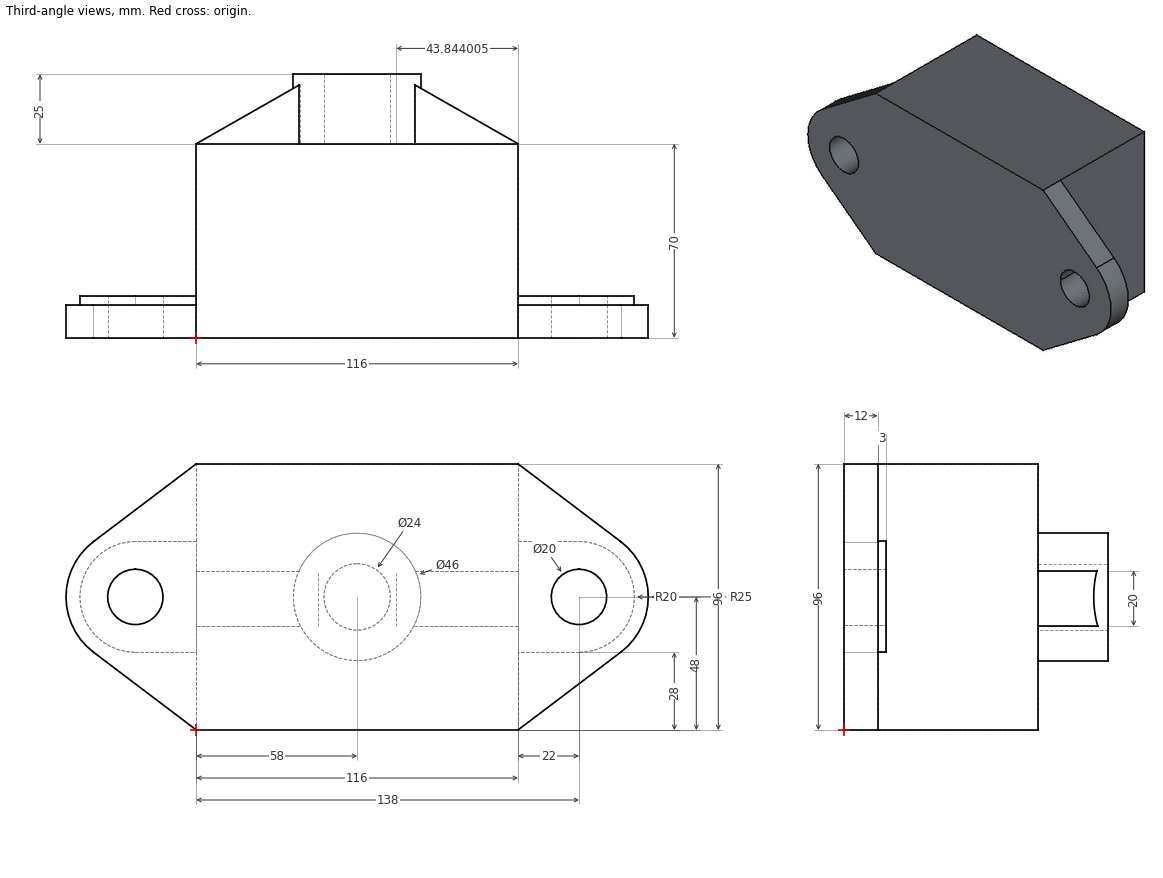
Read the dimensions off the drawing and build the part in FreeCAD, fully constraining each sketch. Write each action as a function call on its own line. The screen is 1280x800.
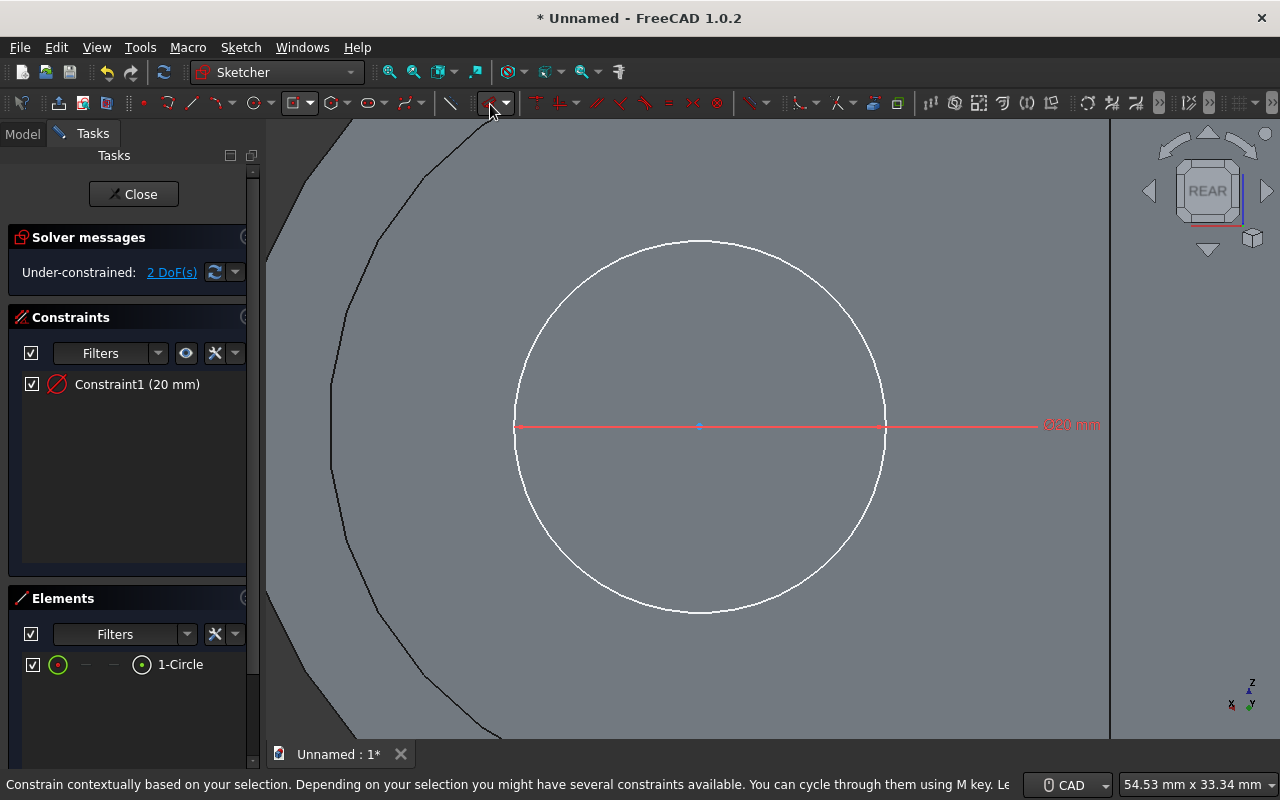
click(700, 427)
click(666, 569)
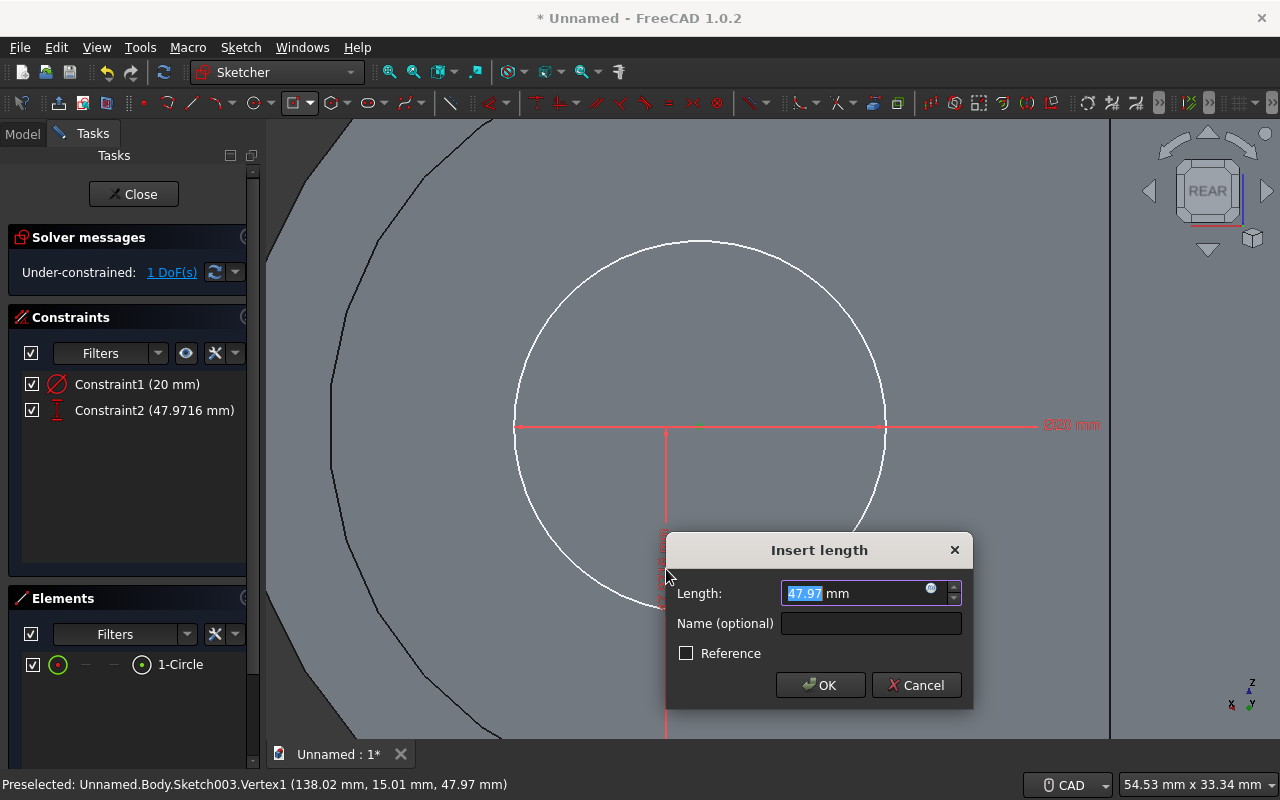
text(48)
key(Return)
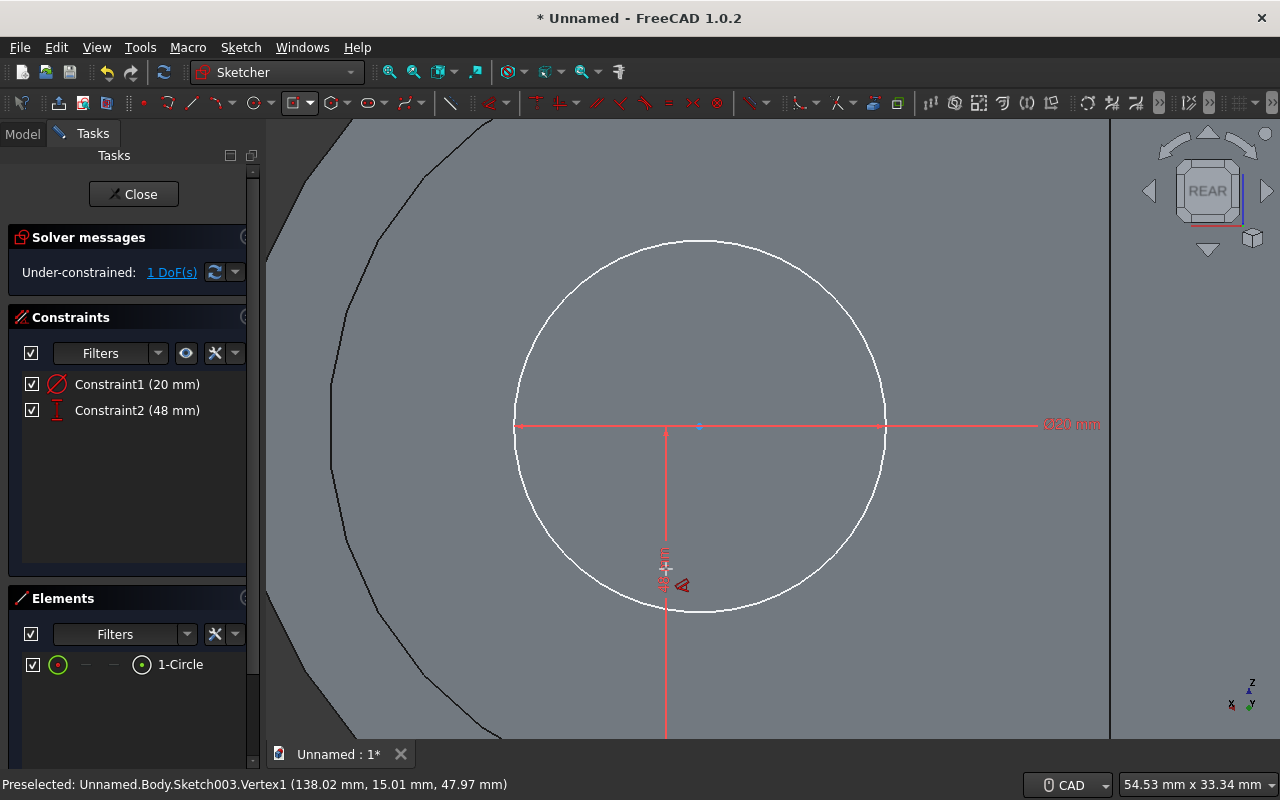
click(700, 426)
click(908, 392)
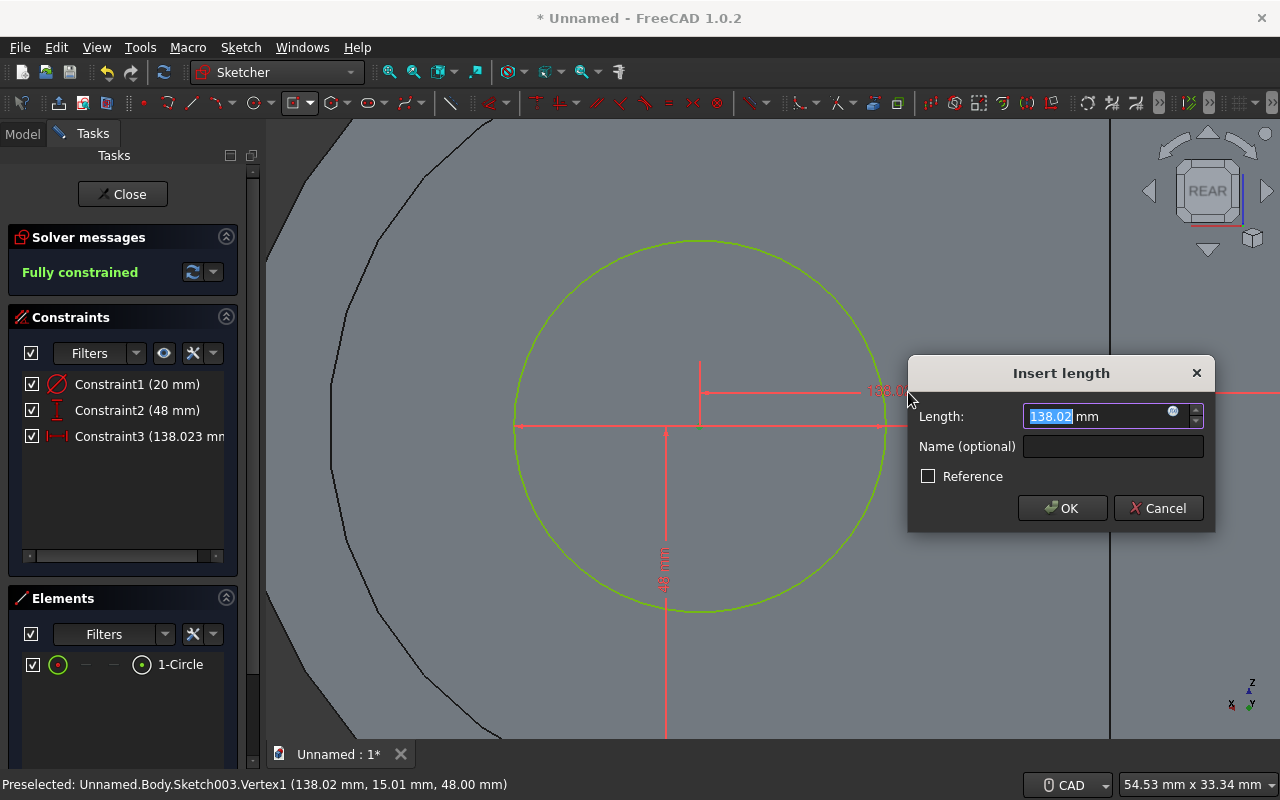
text(138)
key(Return)
key(Escape)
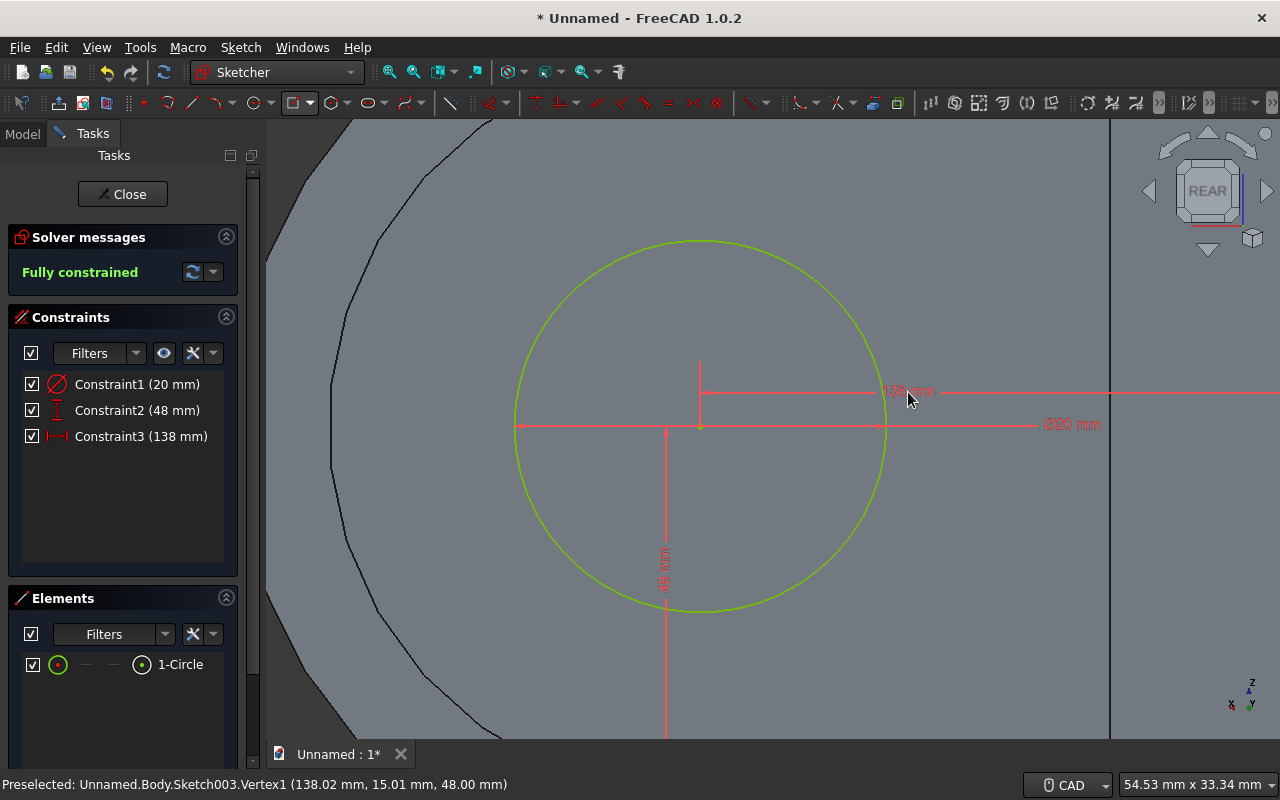
click(123, 194)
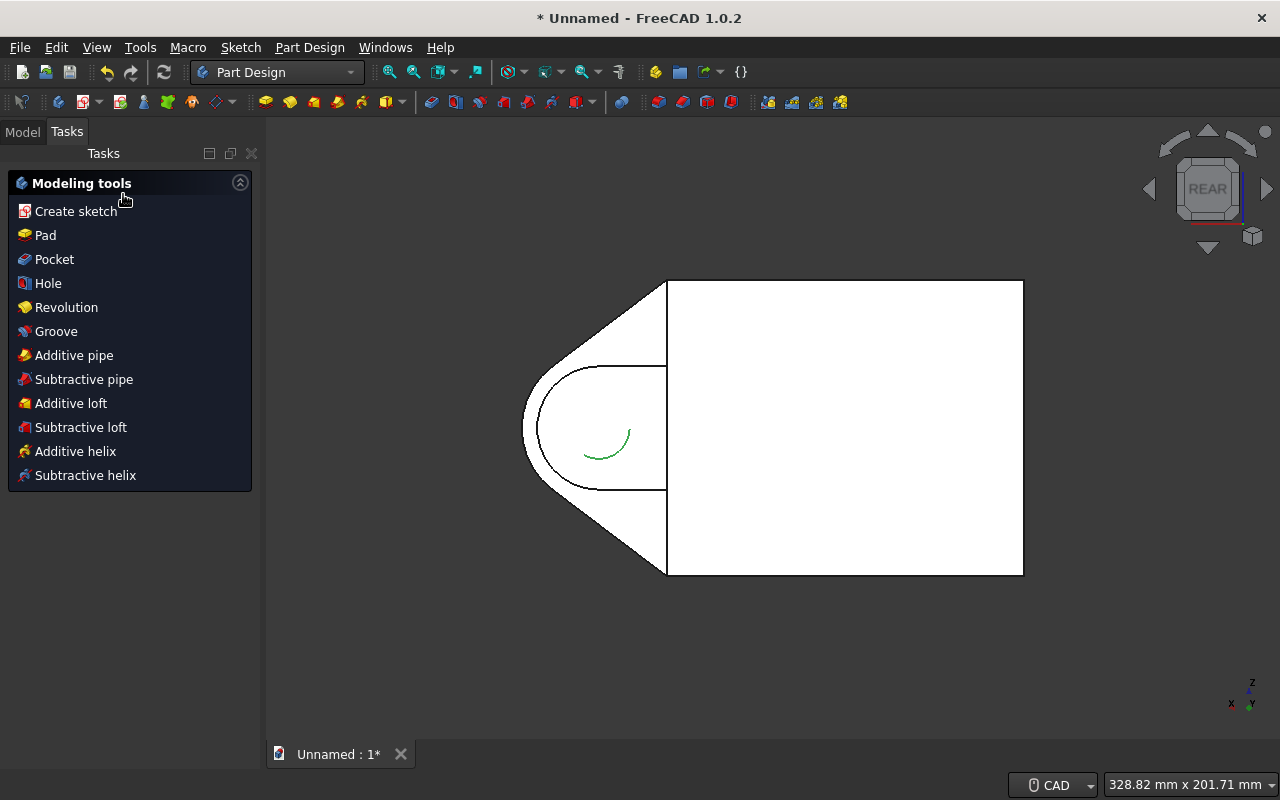
click(432, 102)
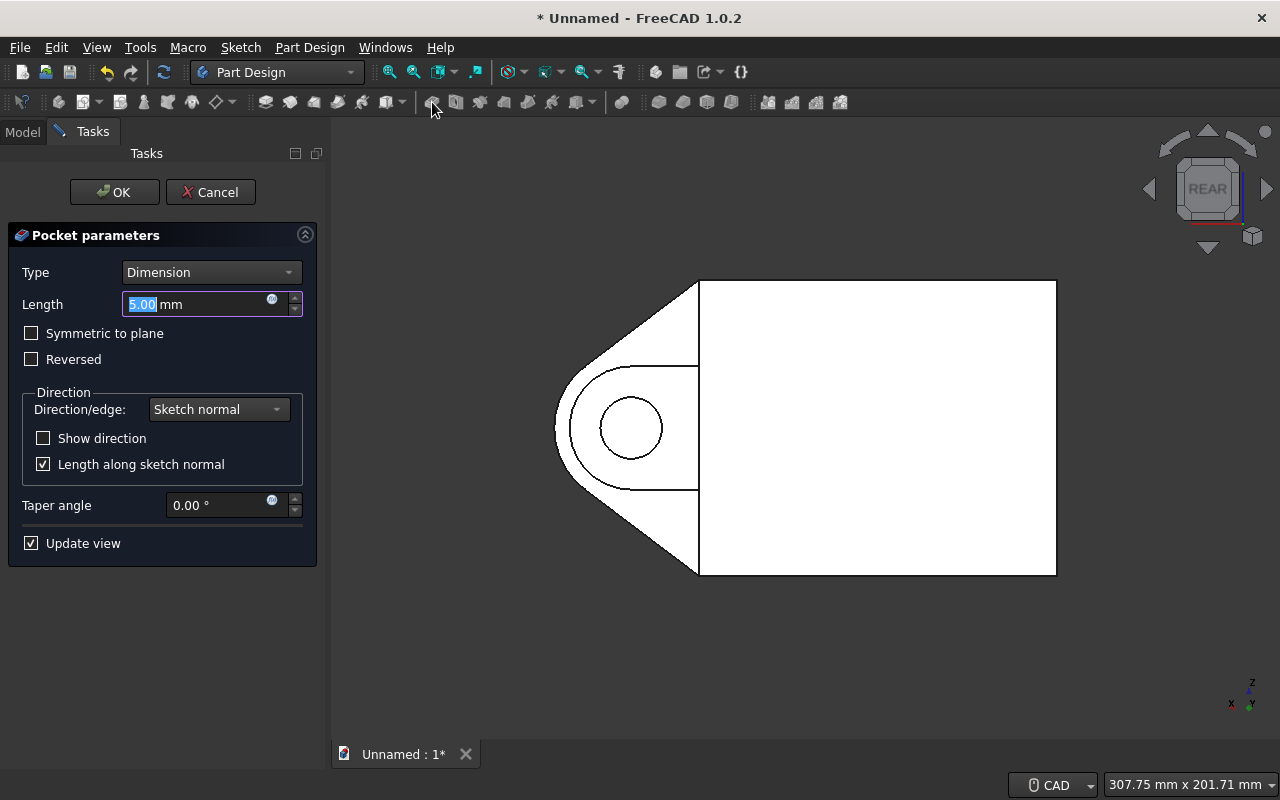
click(212, 272)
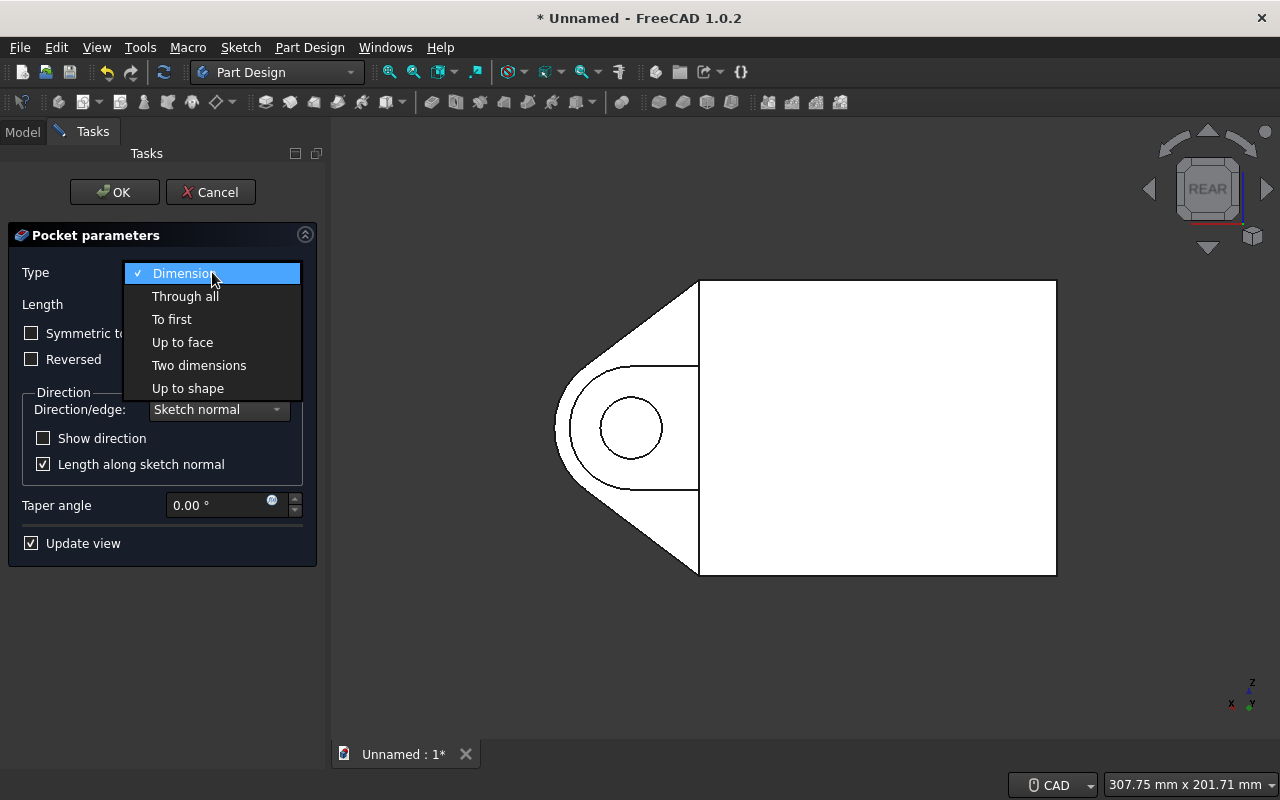
click(212, 296)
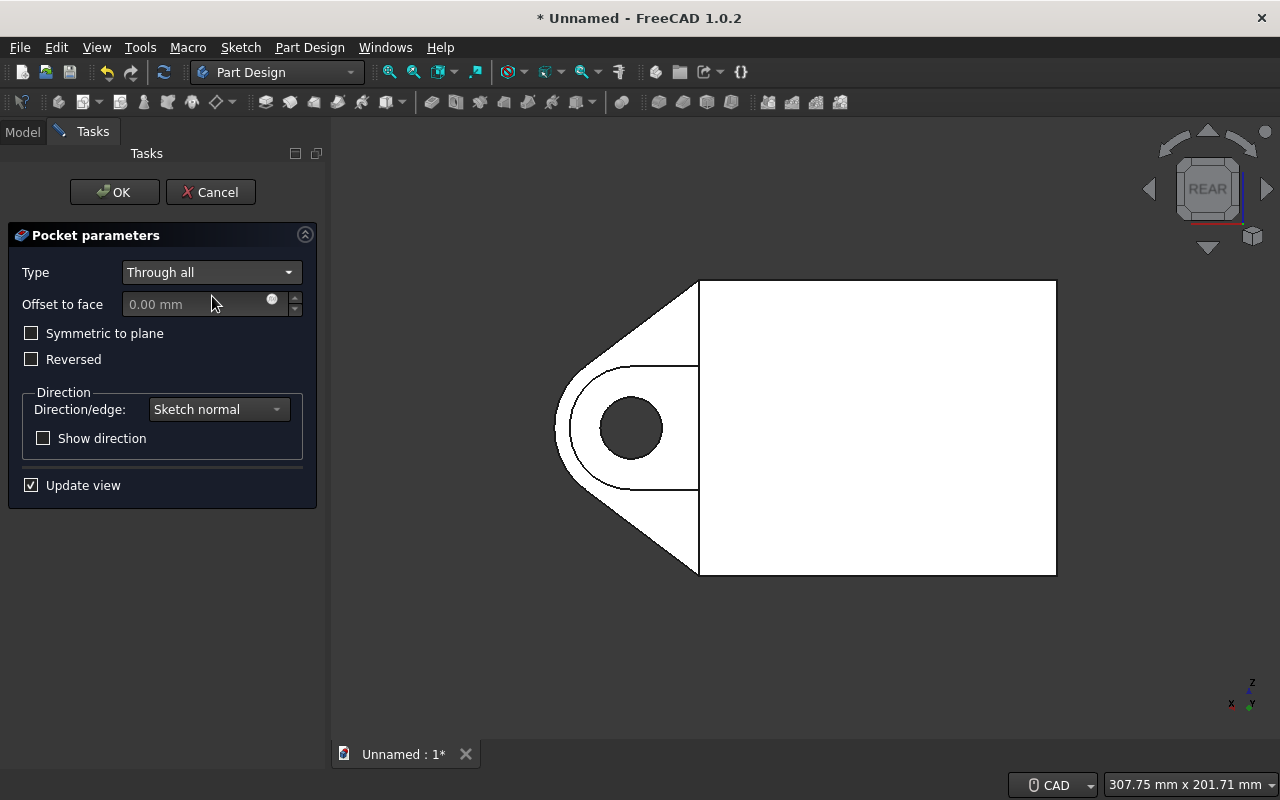
click(115, 192)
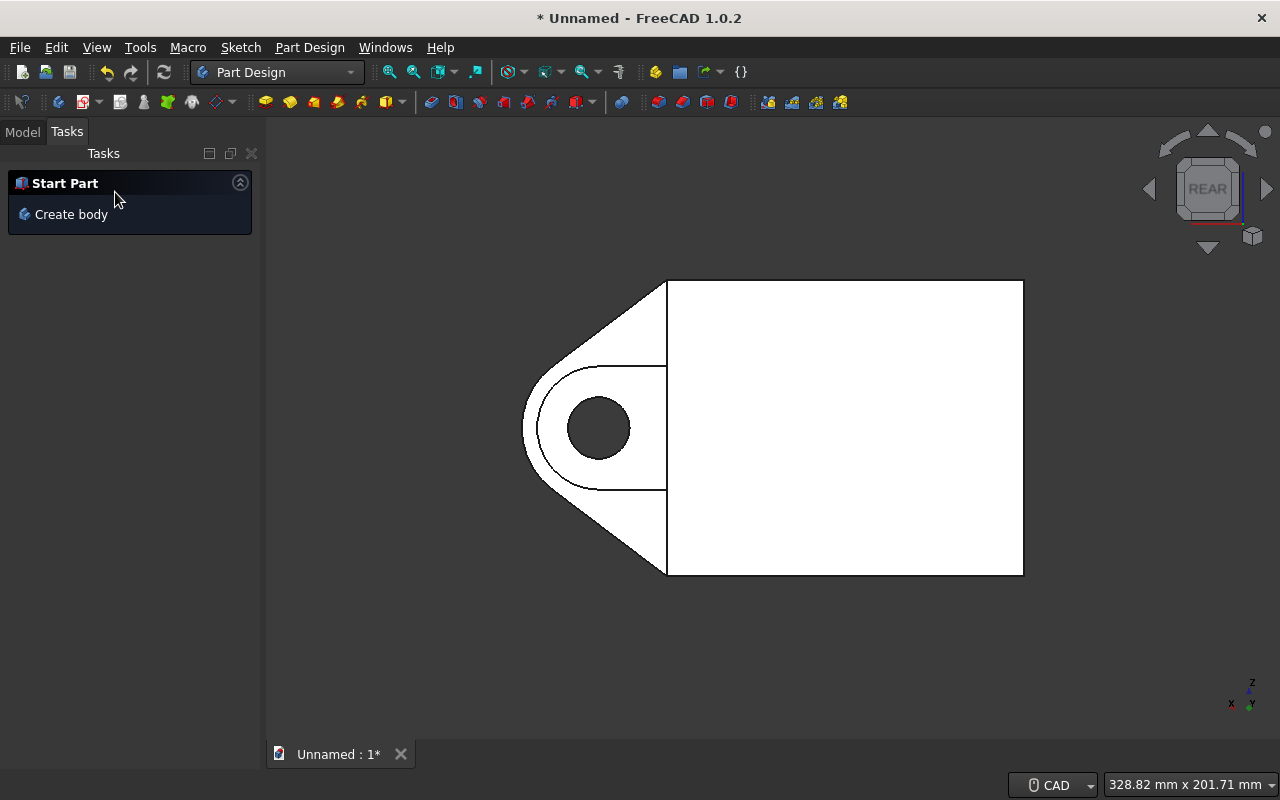
click(23, 131)